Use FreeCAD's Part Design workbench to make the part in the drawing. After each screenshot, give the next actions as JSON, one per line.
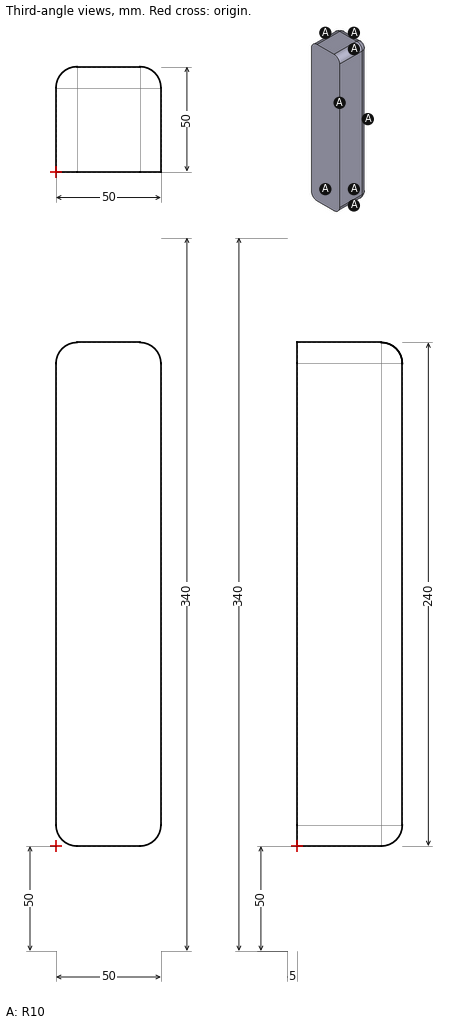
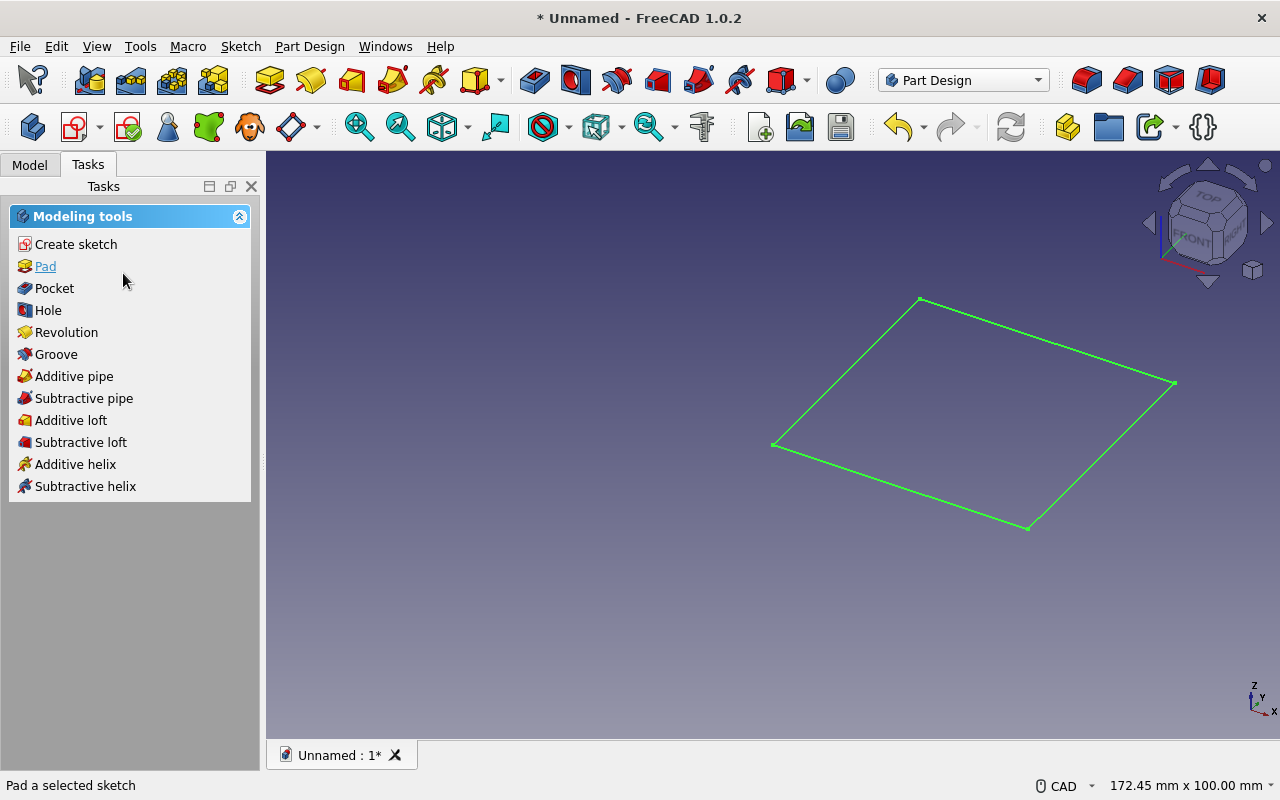
{"action": "left_click", "coordinate": [270, 80]}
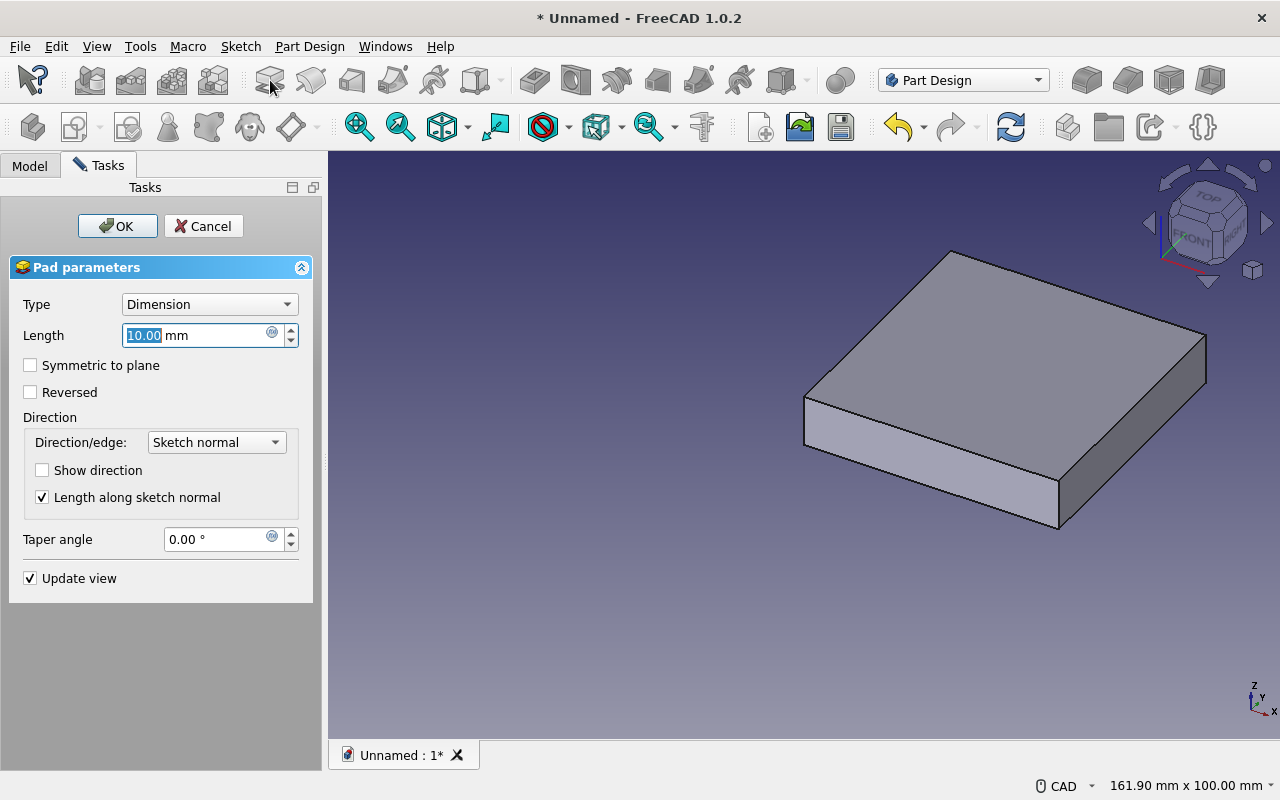
{"action": "type", "text": "240"}
{"action": "key", "text": "Tab"}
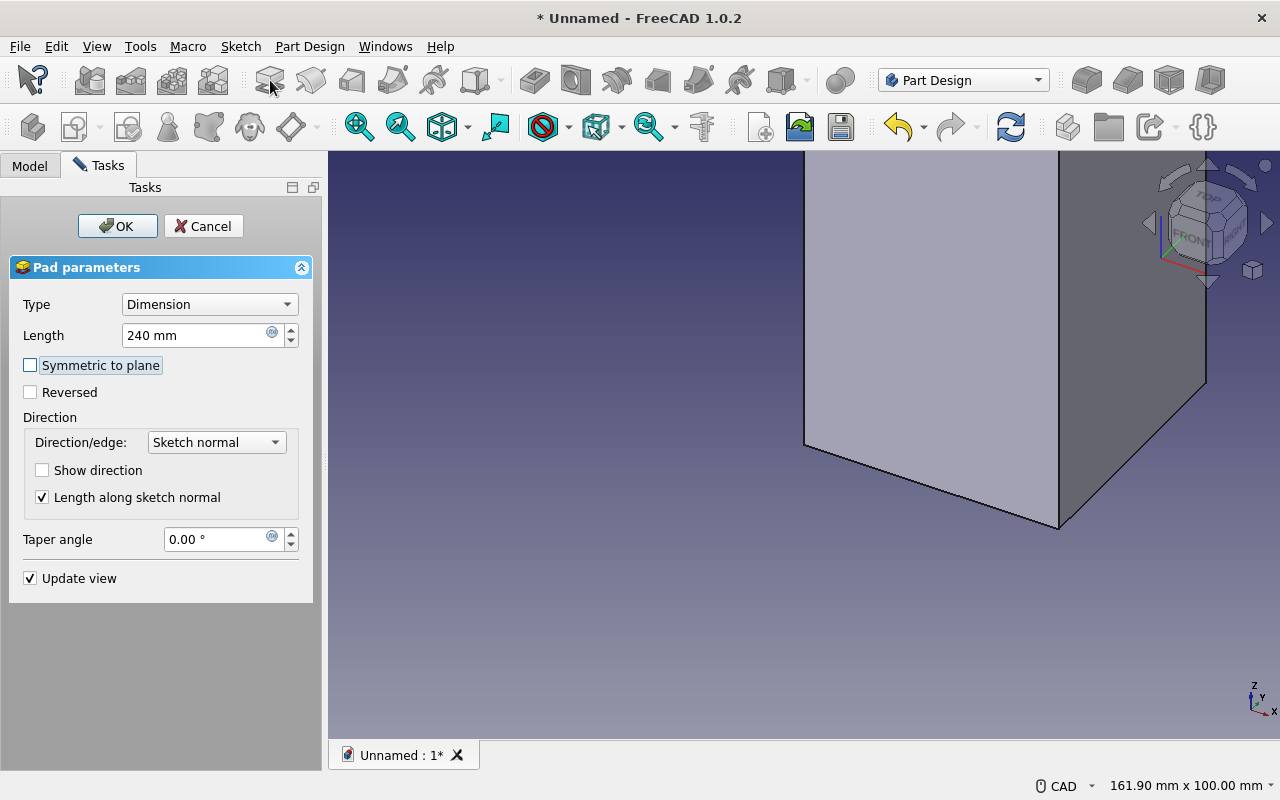
{"action": "left_click", "coordinate": [118, 226]}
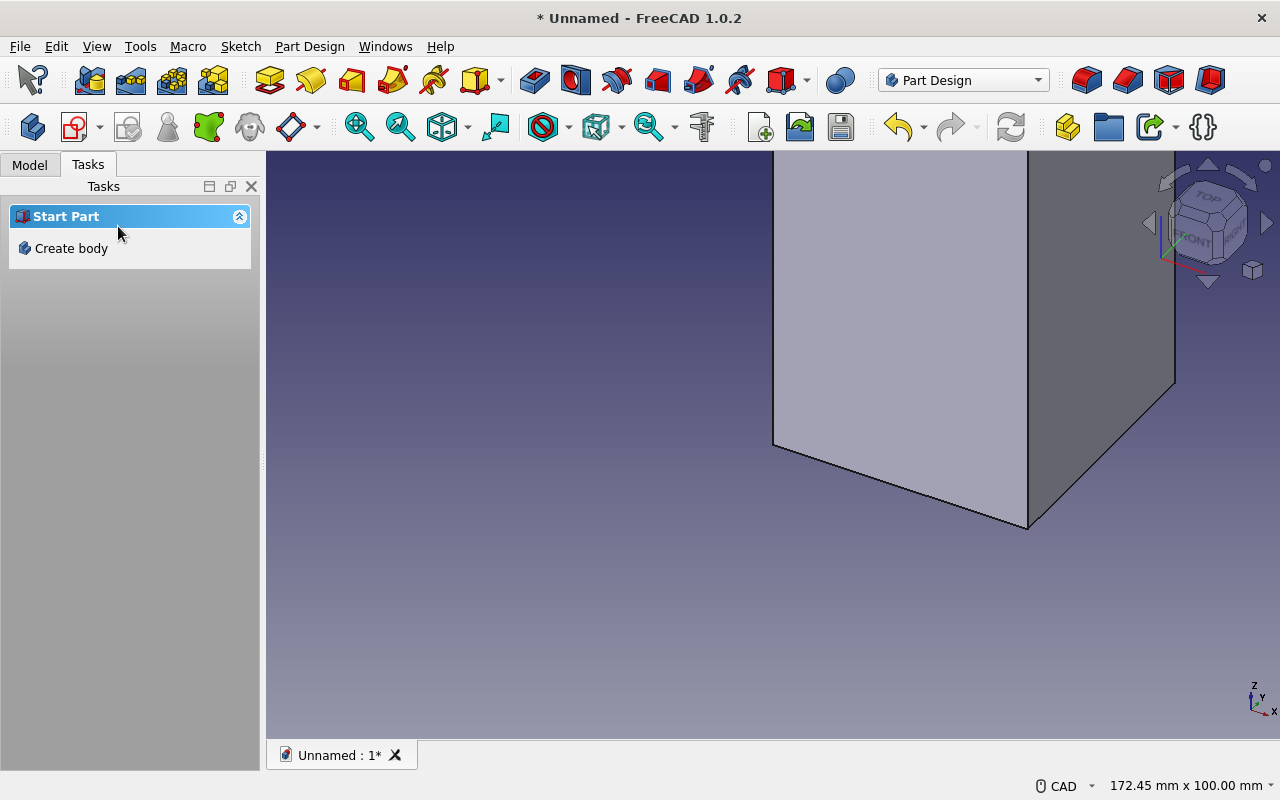
{"action": "key", "text": "v f"}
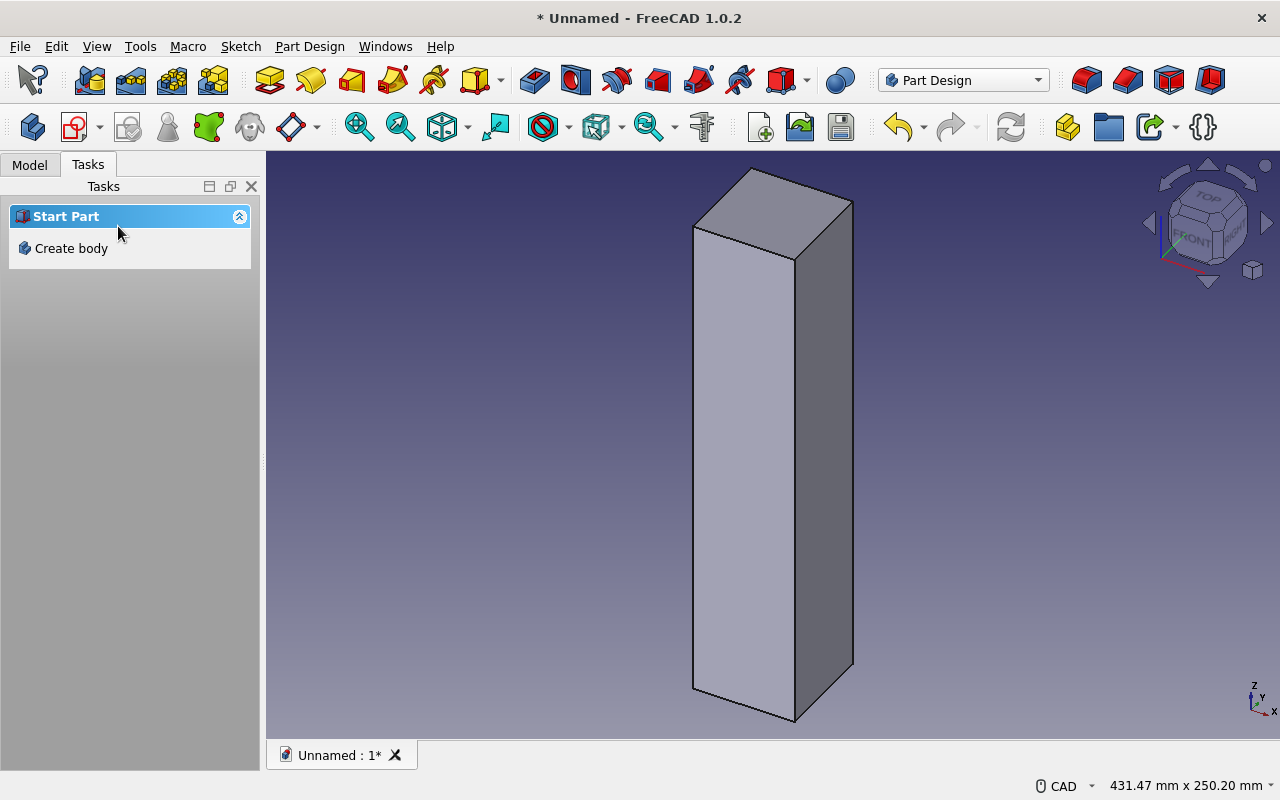
{"action": "left_click", "coordinate": [744, 341]}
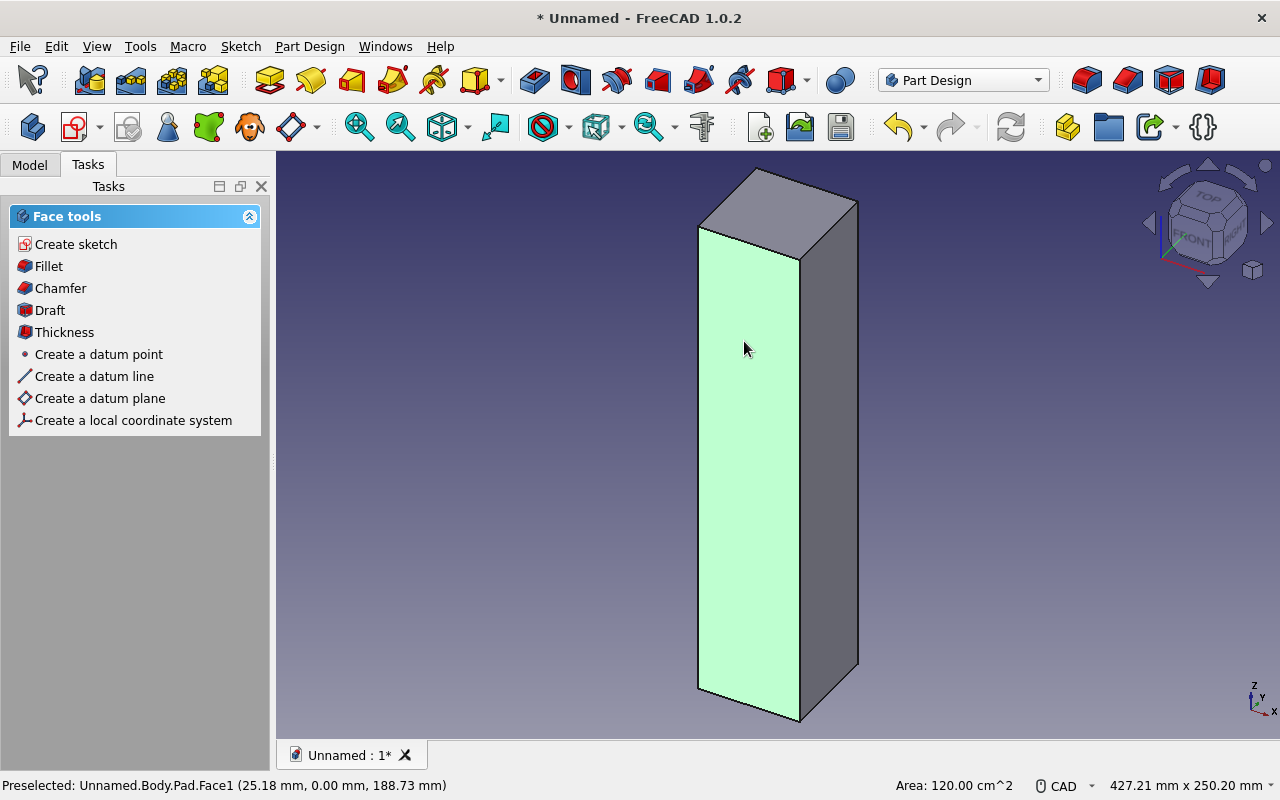
{"action": "left_click", "coordinate": [74, 128]}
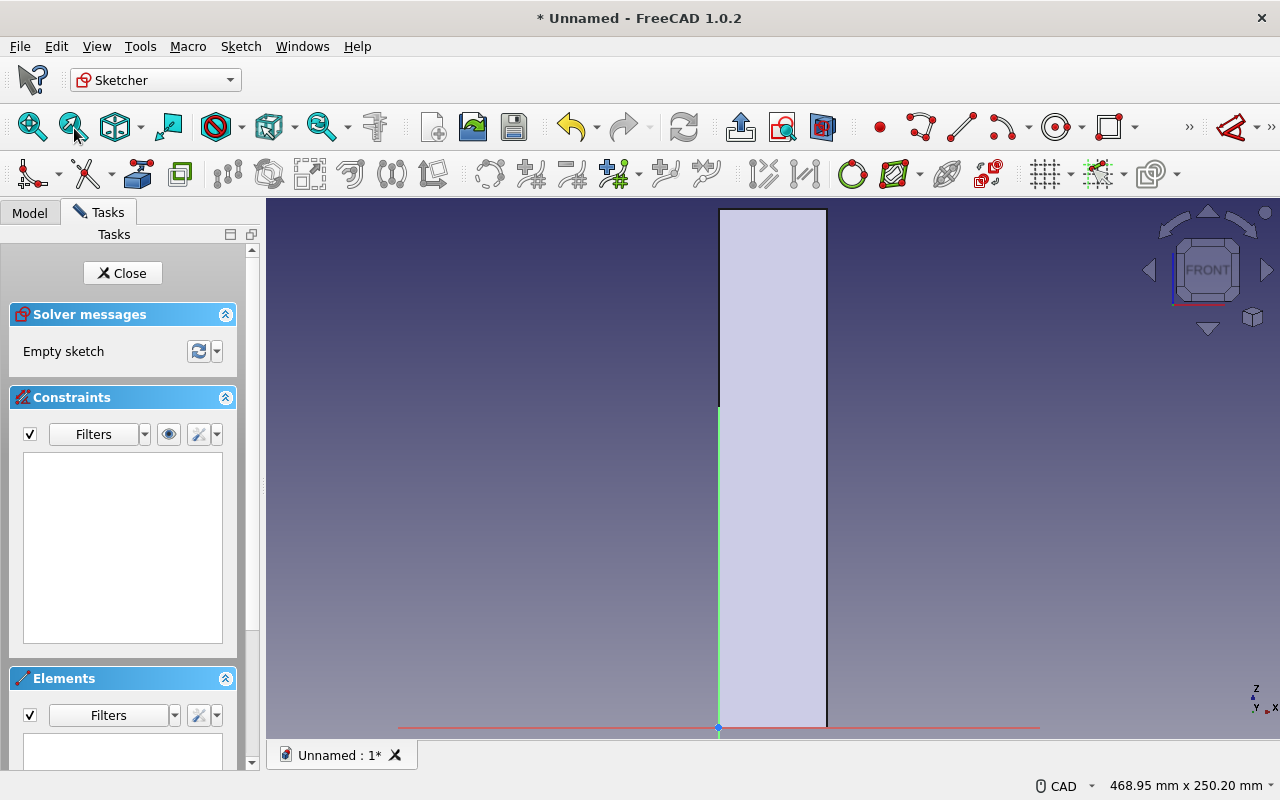
{"action": "scroll", "coordinate": [649, 468], "scroll_direction": "down", "scroll_amount": 4}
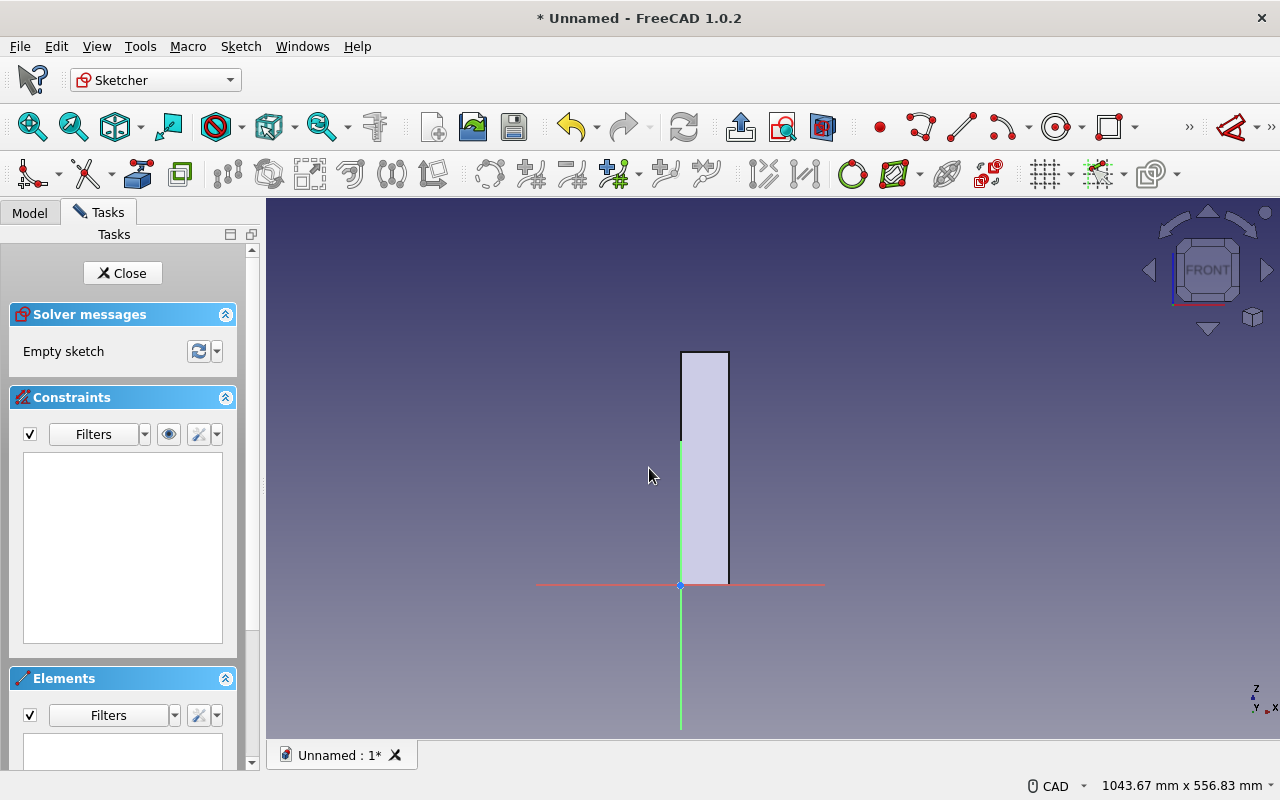
{"action": "key", "text": "g r"}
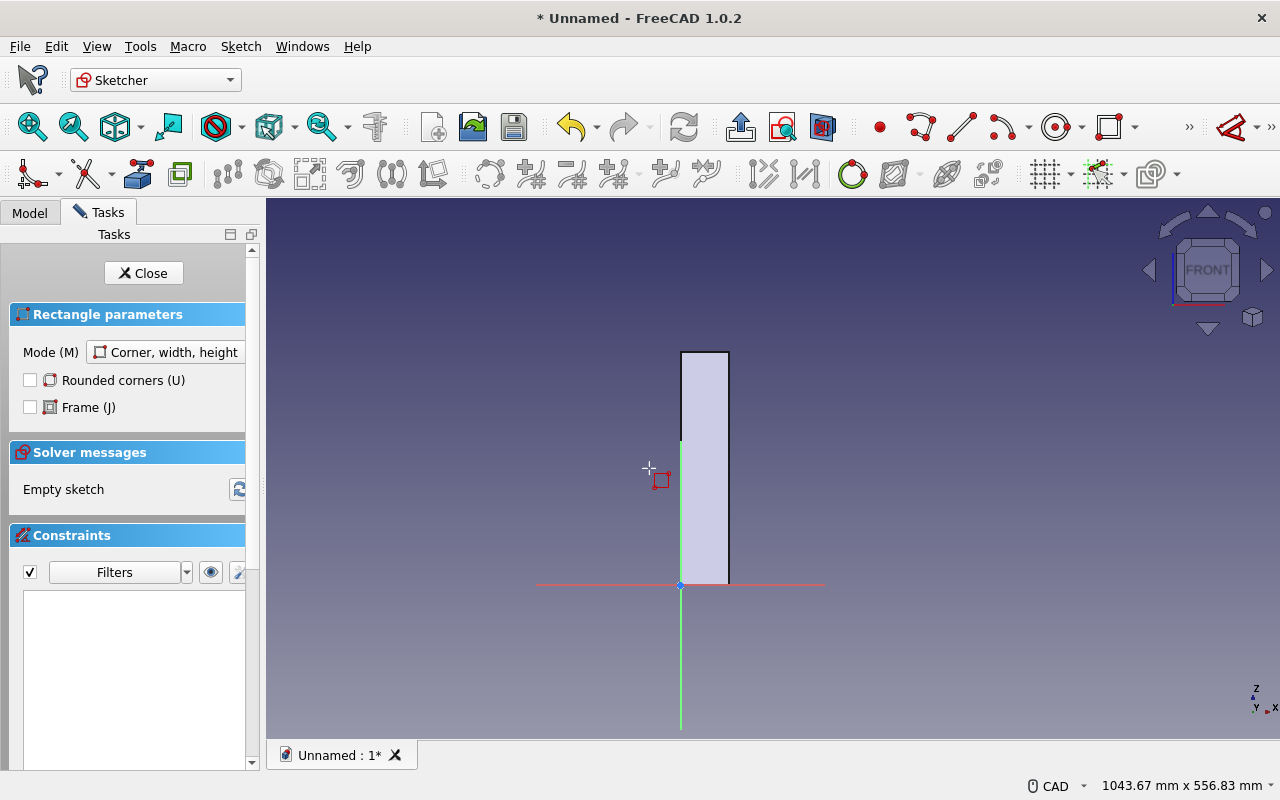
{"action": "left_click", "coordinate": [681, 303]}
{"action": "mouse_move", "coordinate": [729, 634]}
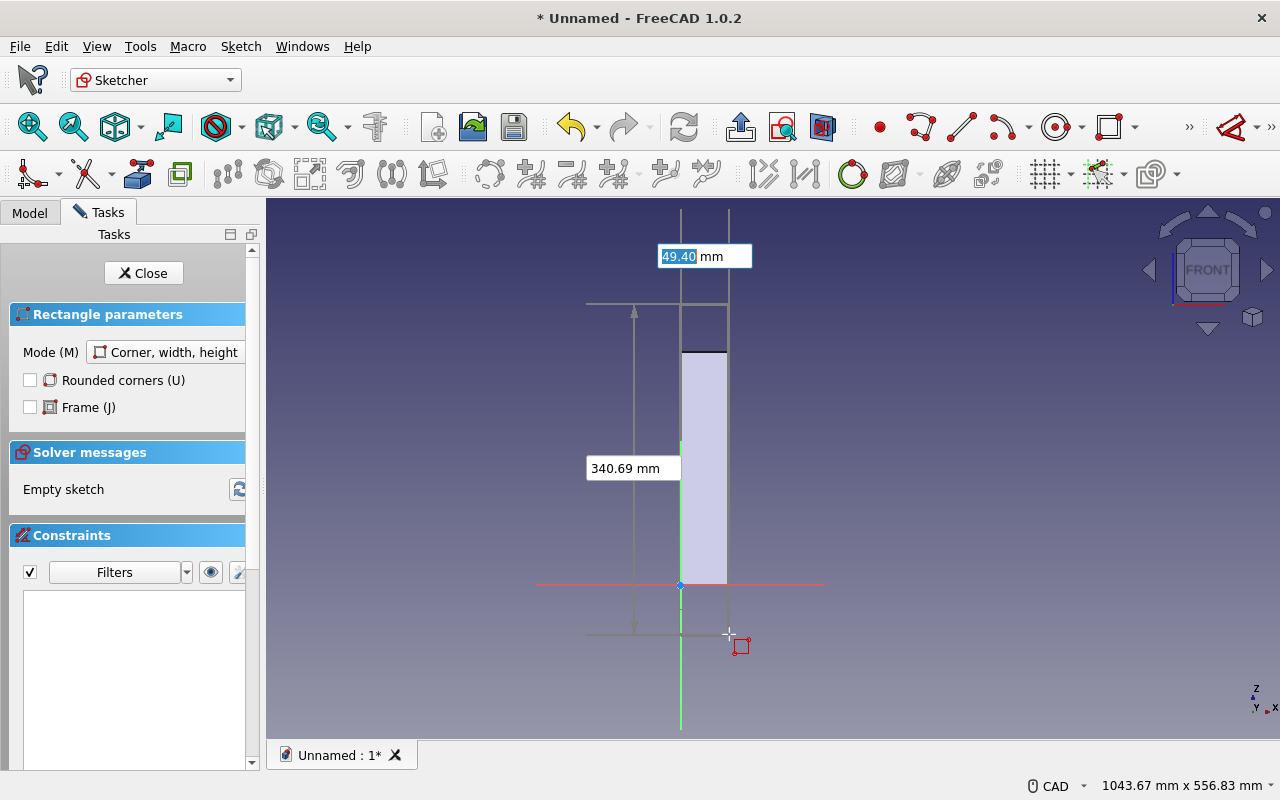
{"action": "type", "text": "50"}
{"action": "key", "text": "Tab"}
{"action": "type", "text": "340"}
{"action": "key", "text": "Return"}
{"action": "key", "text": "Escape"}